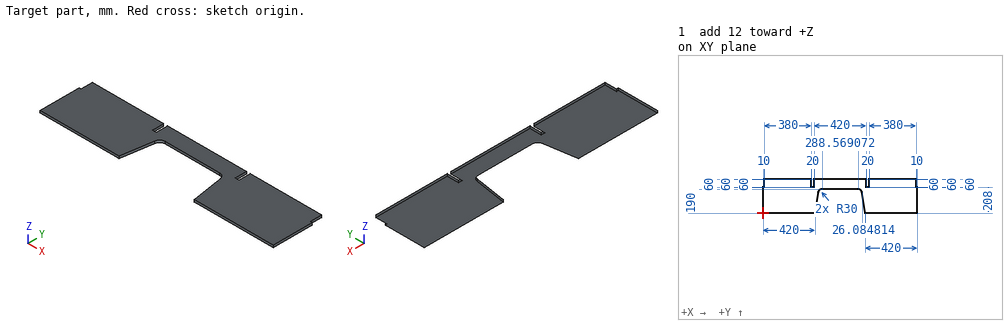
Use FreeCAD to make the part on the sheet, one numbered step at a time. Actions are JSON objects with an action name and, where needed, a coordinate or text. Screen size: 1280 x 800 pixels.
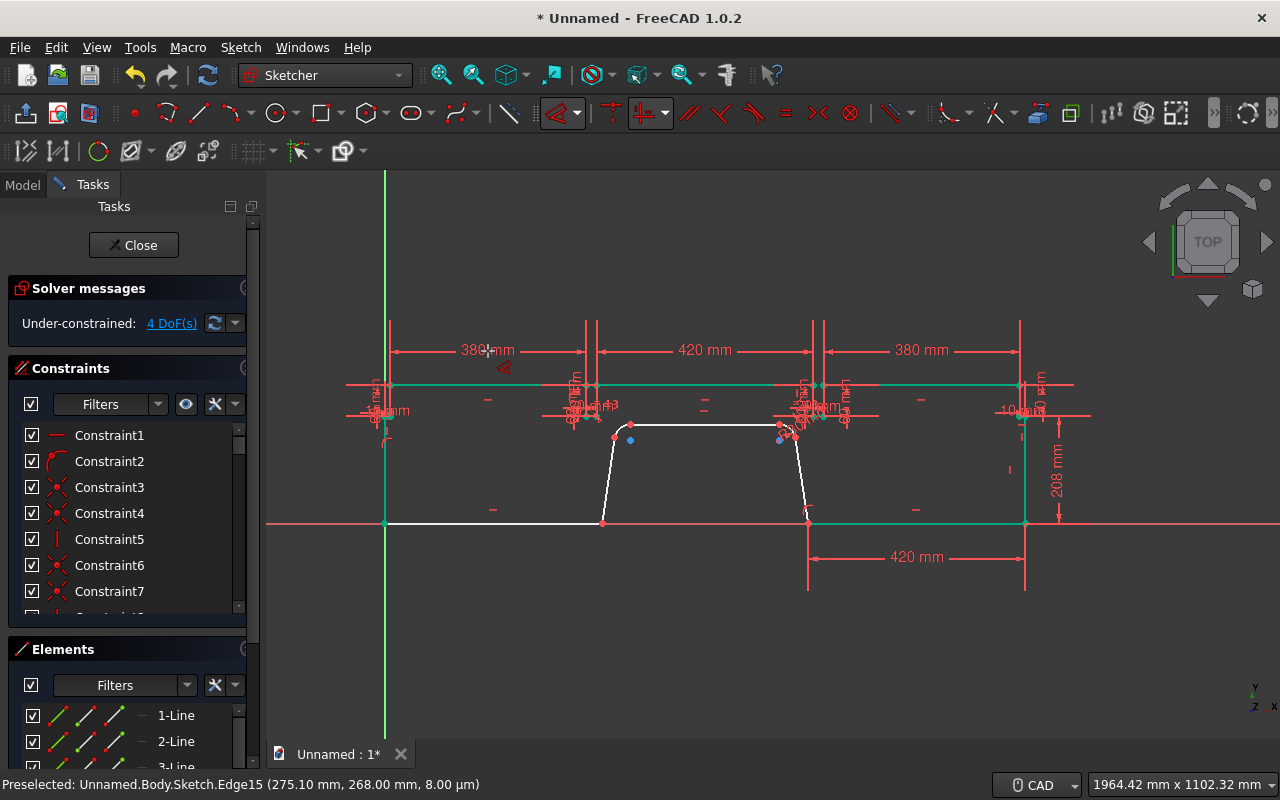
{"action": "left_click", "coordinate": [450, 524]}
{"action": "left_click", "coordinate": [494, 558]}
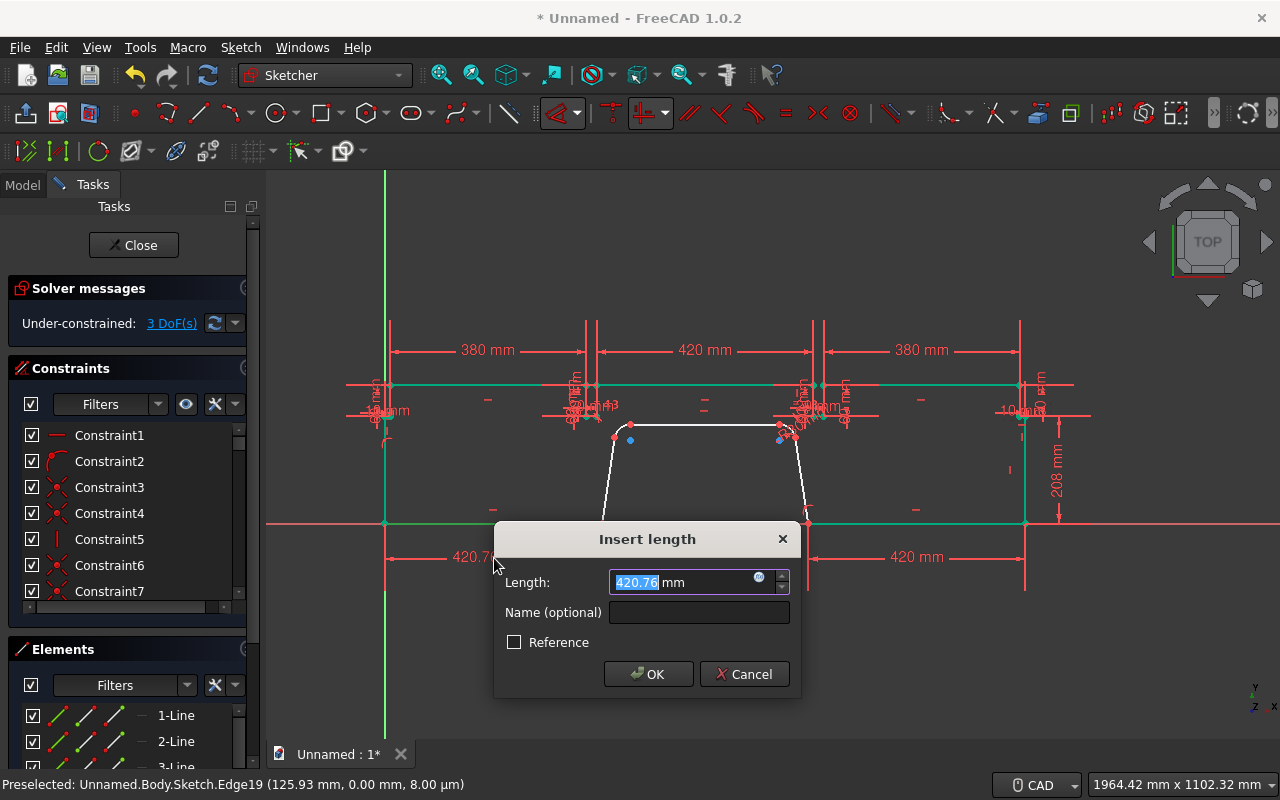
{"action": "type", "text": "420"}
{"action": "key", "text": "Return"}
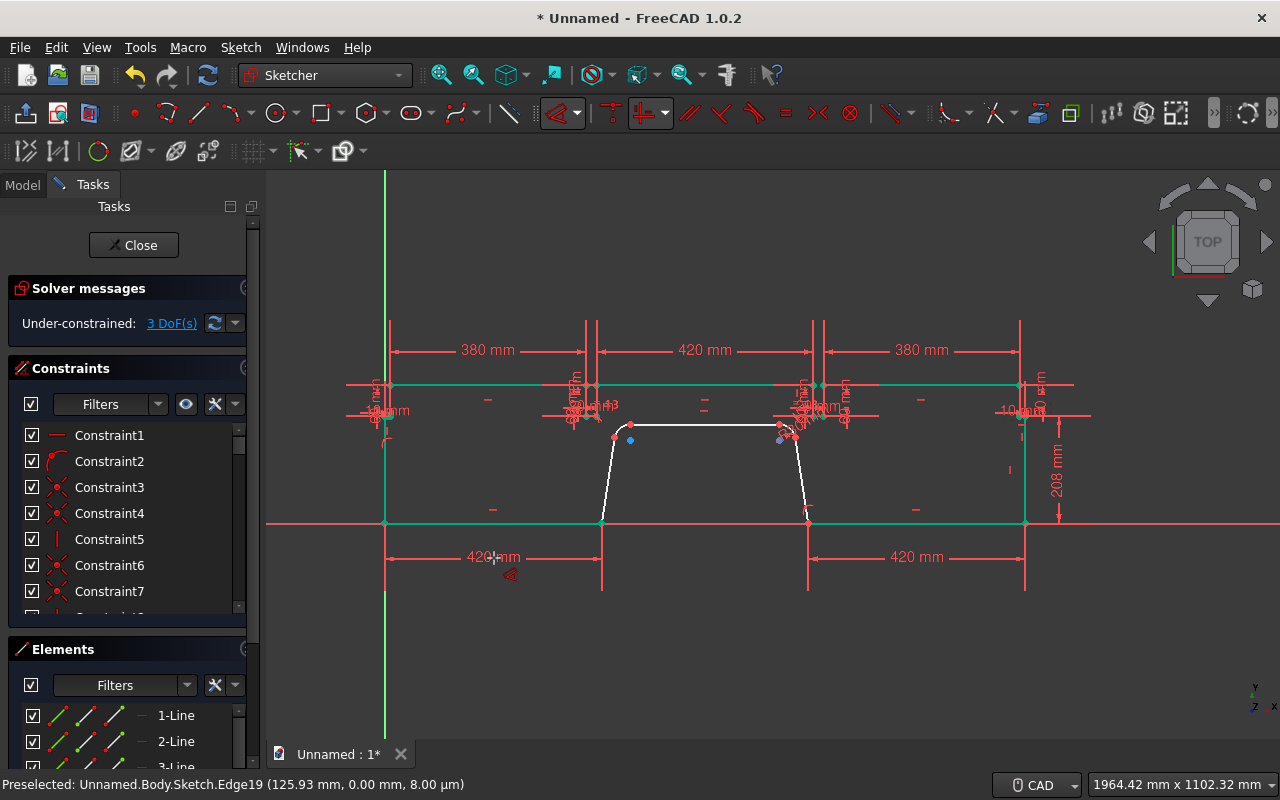
{"action": "left_click", "coordinate": [630, 425]}
{"action": "left_click", "coordinate": [351, 474]}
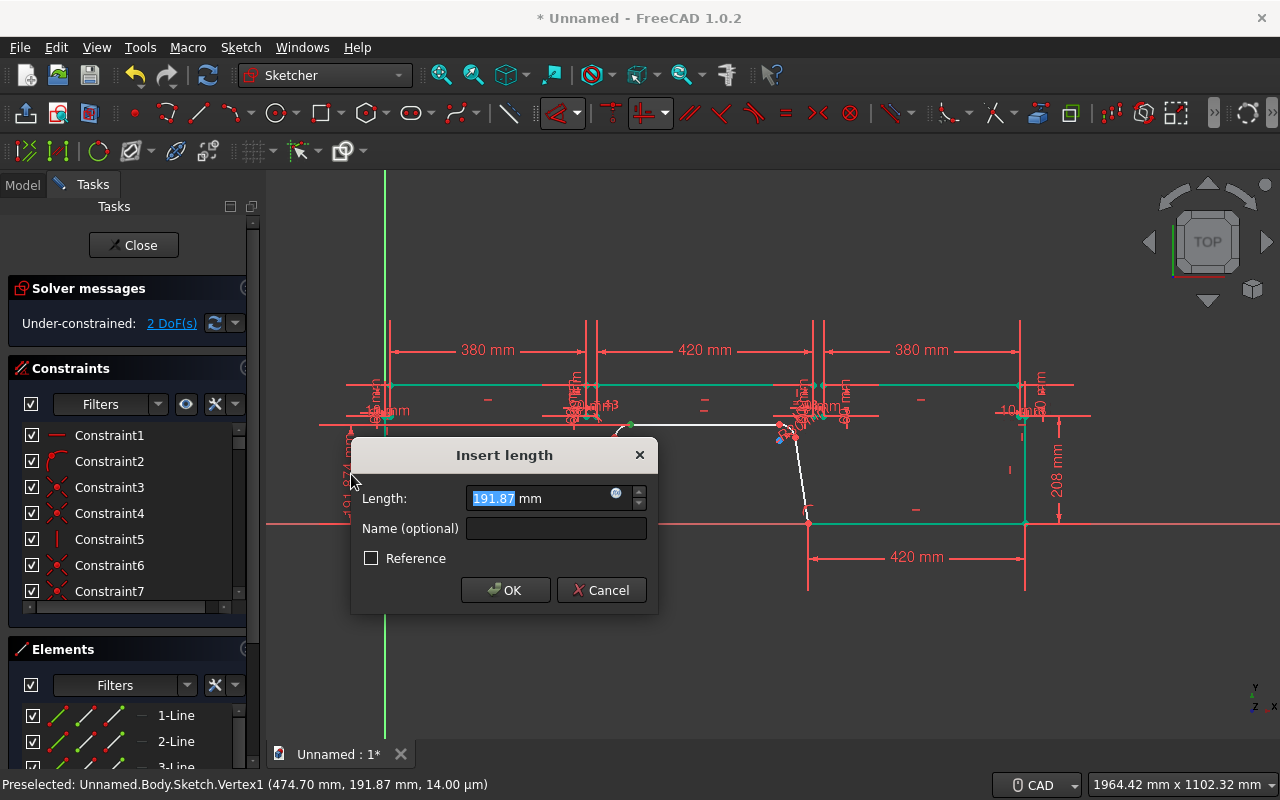
{"action": "type", "text": "190"}
{"action": "key", "text": "Return"}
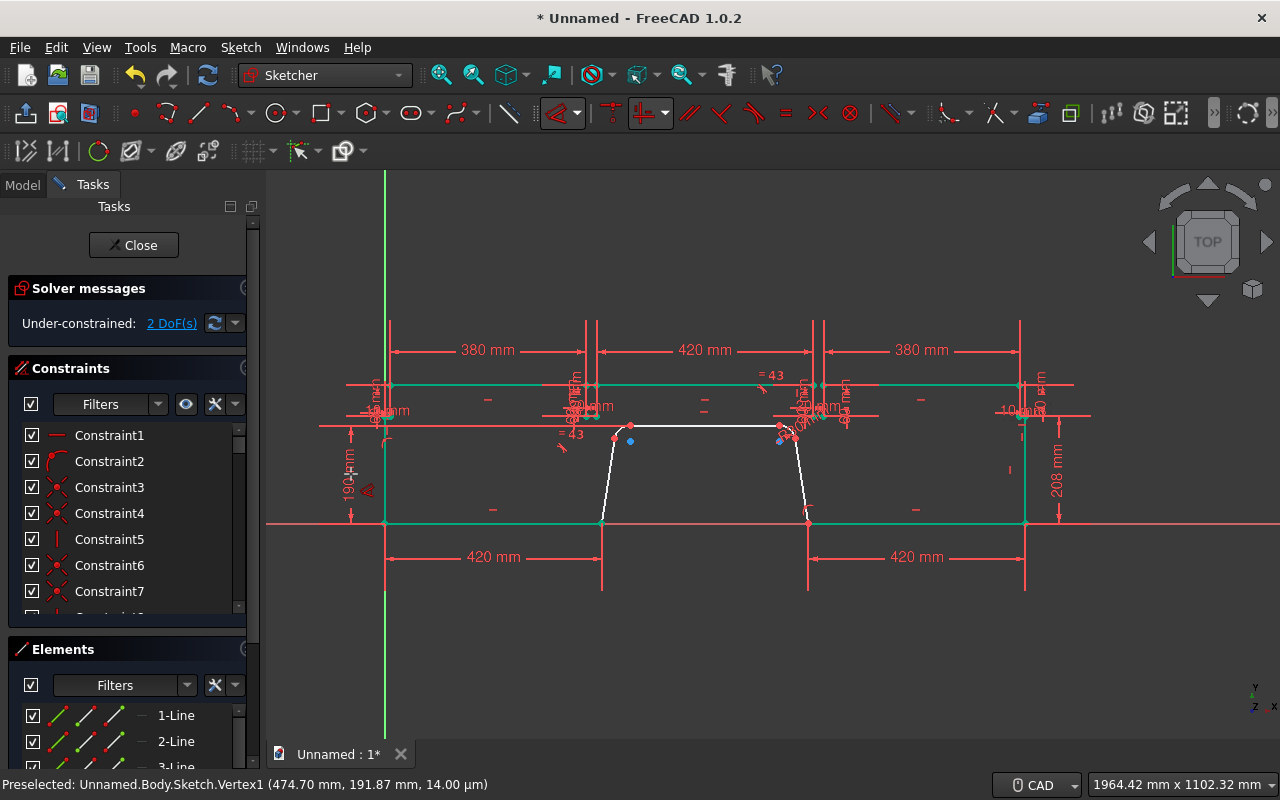
{"action": "left_click", "coordinate": [675, 426]}
{"action": "left_click", "coordinate": [705, 460]}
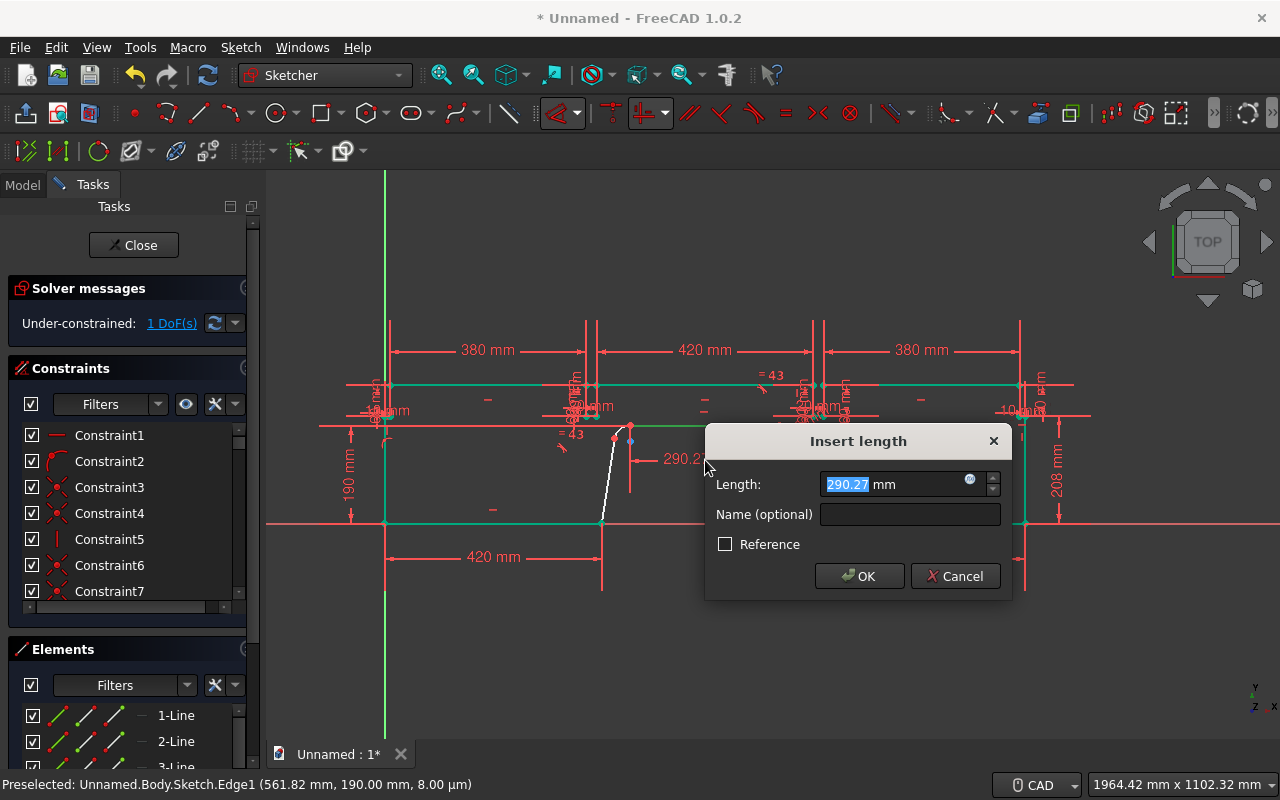
{"action": "type", "text": "288.569072"}
{"action": "key", "text": "Return"}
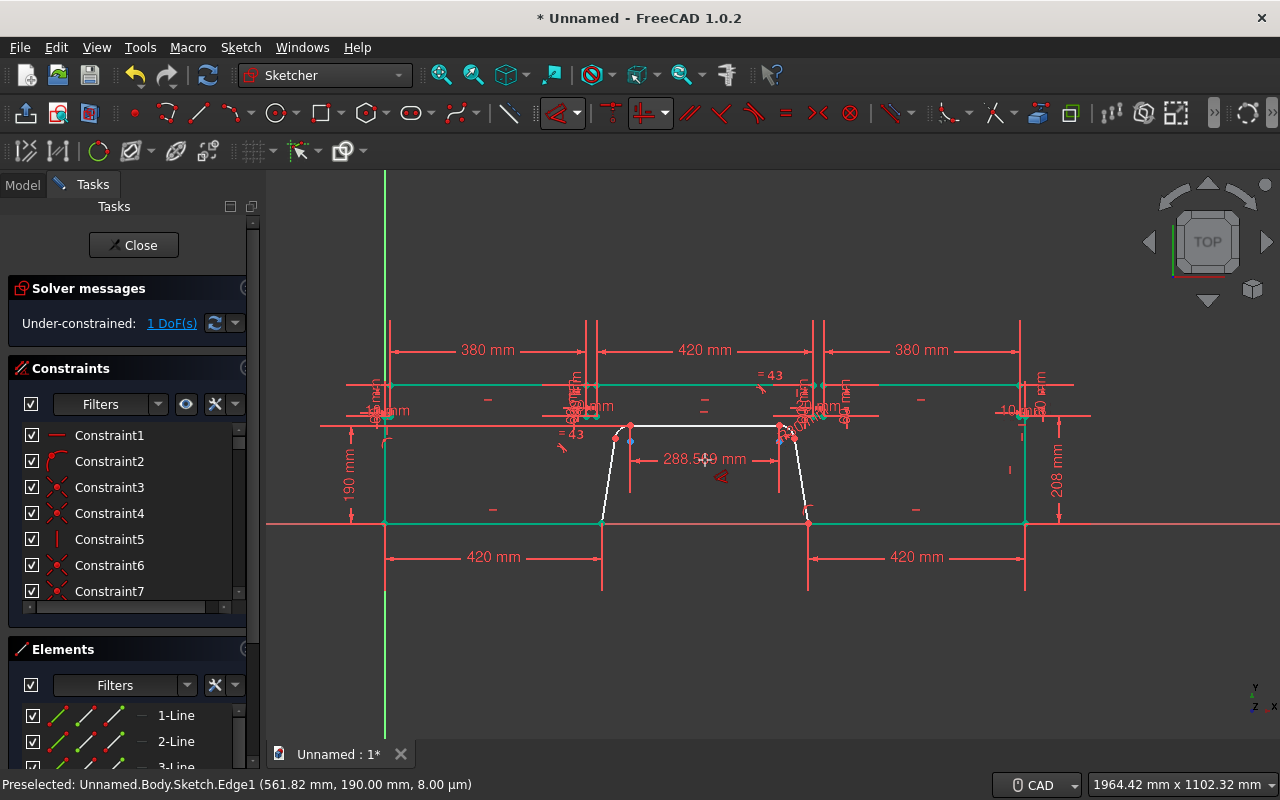
{"action": "scroll", "coordinate": [799, 464], "scroll_direction": "up", "scroll_amount": 6}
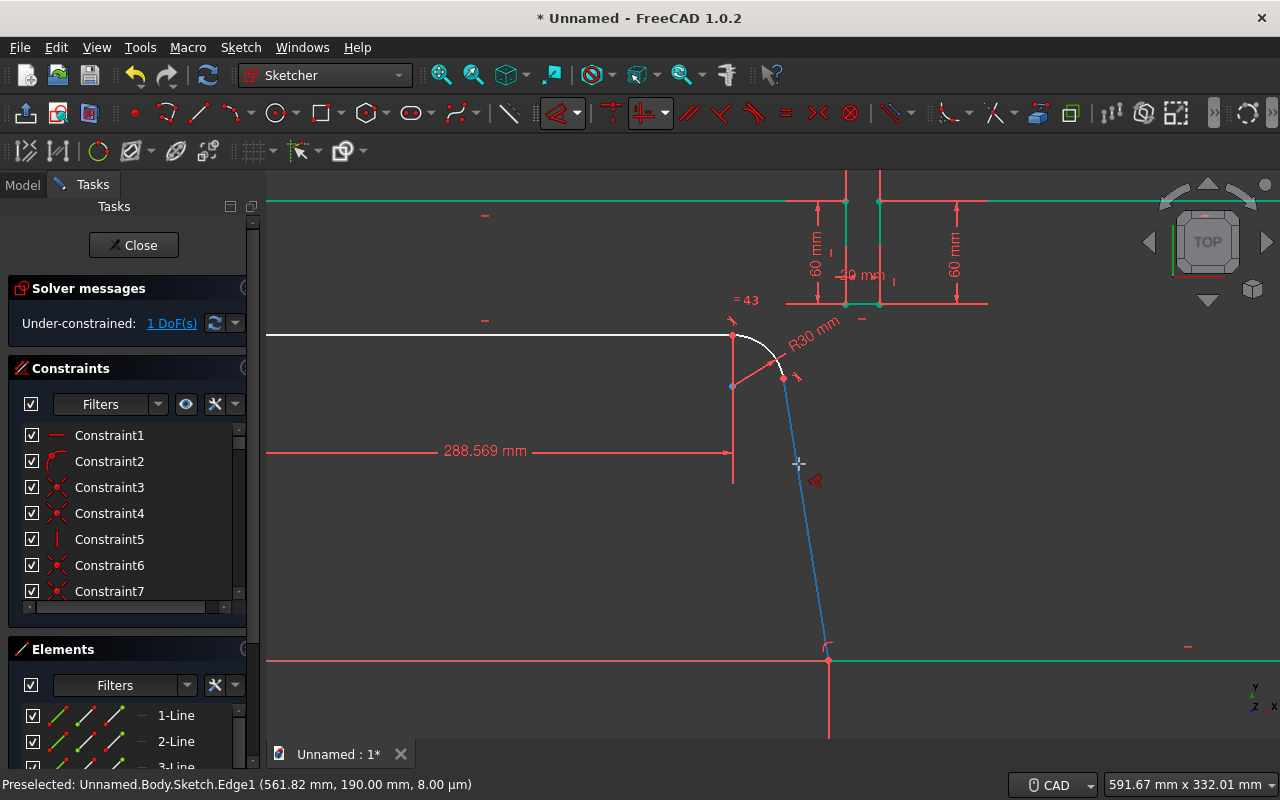
{"action": "left_click", "coordinate": [797, 463]}
{"action": "left_click", "coordinate": [806, 695]}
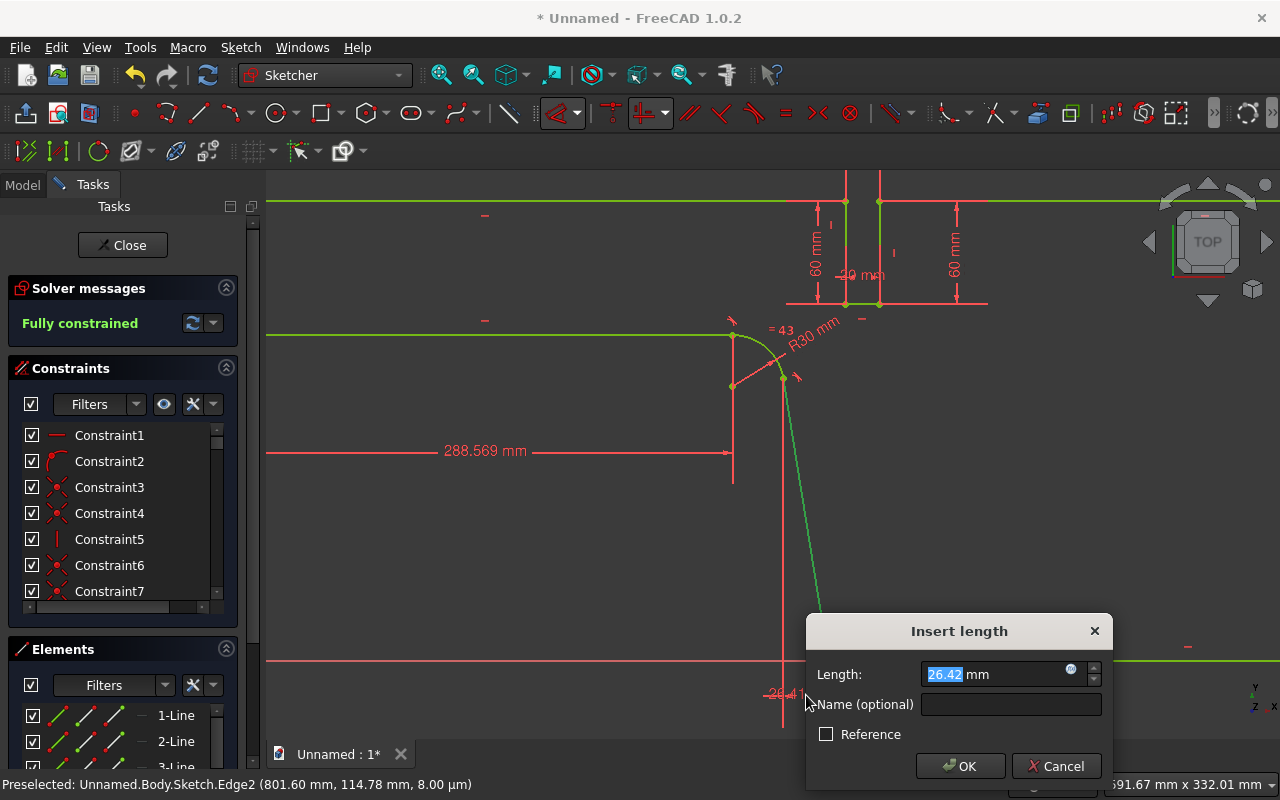
{"action": "type", "text": "26.084814"}
{"action": "key", "text": "Return"}
{"action": "key", "text": "Escape"}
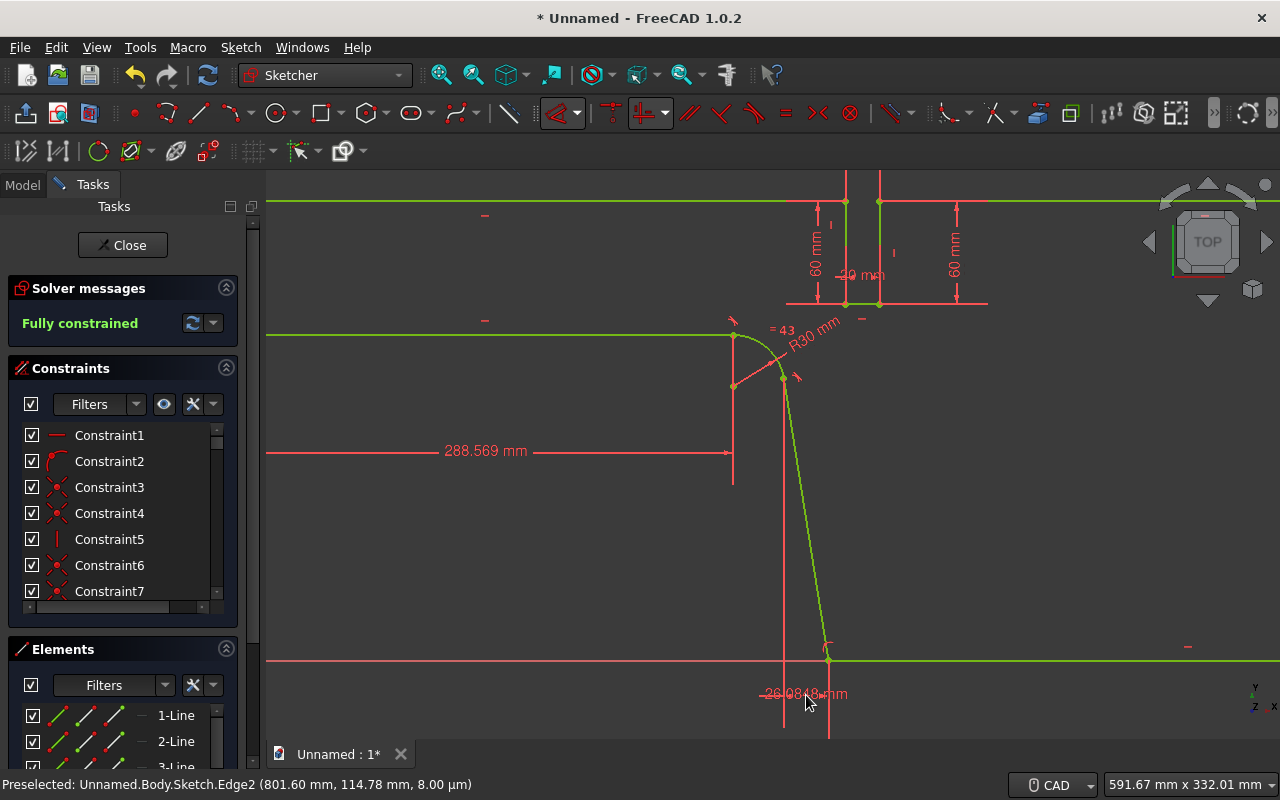
{"action": "left_click", "coordinate": [123, 245]}